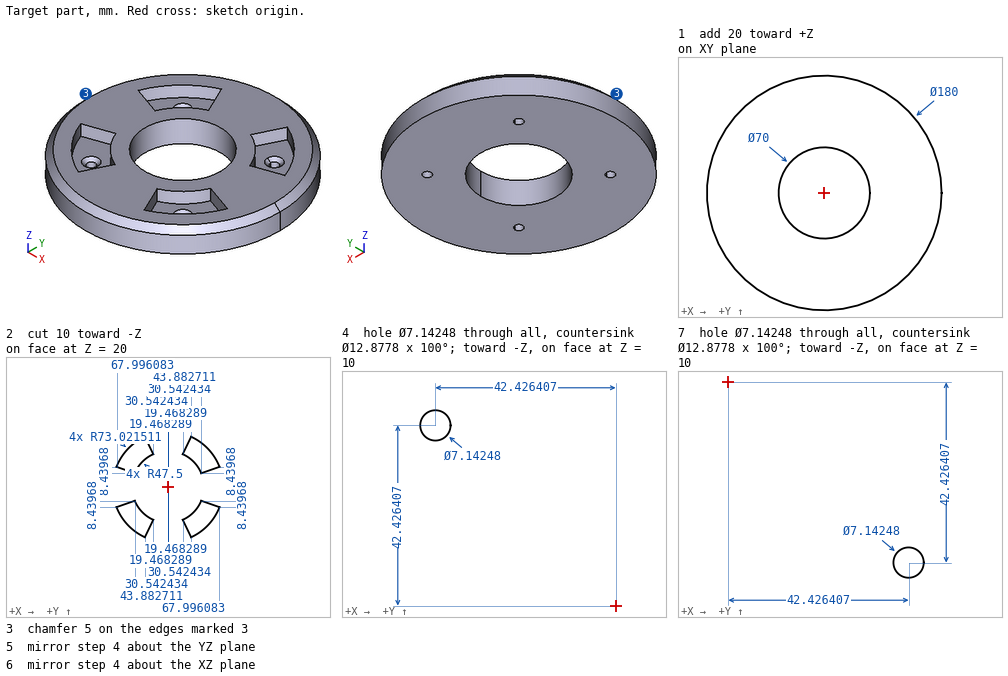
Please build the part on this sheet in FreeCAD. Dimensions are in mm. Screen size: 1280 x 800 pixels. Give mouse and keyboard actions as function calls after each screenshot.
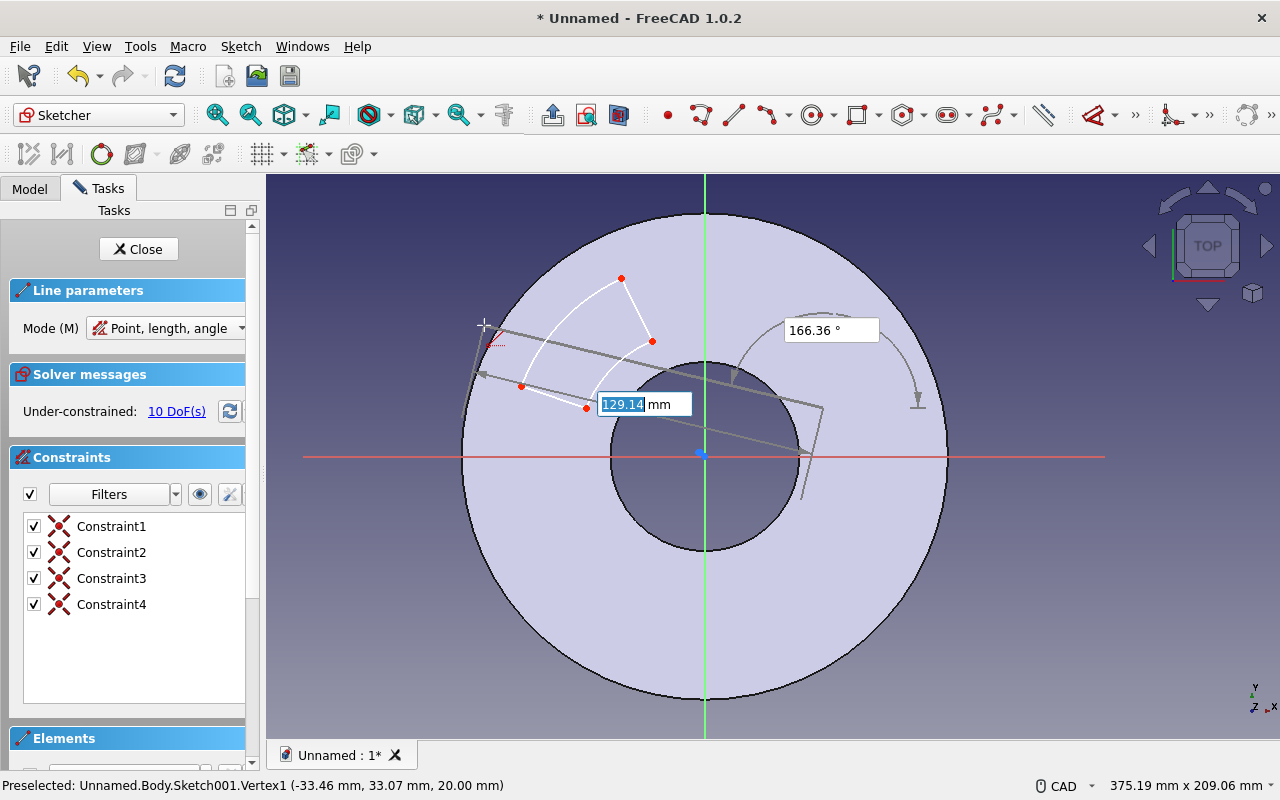
click(889, 385)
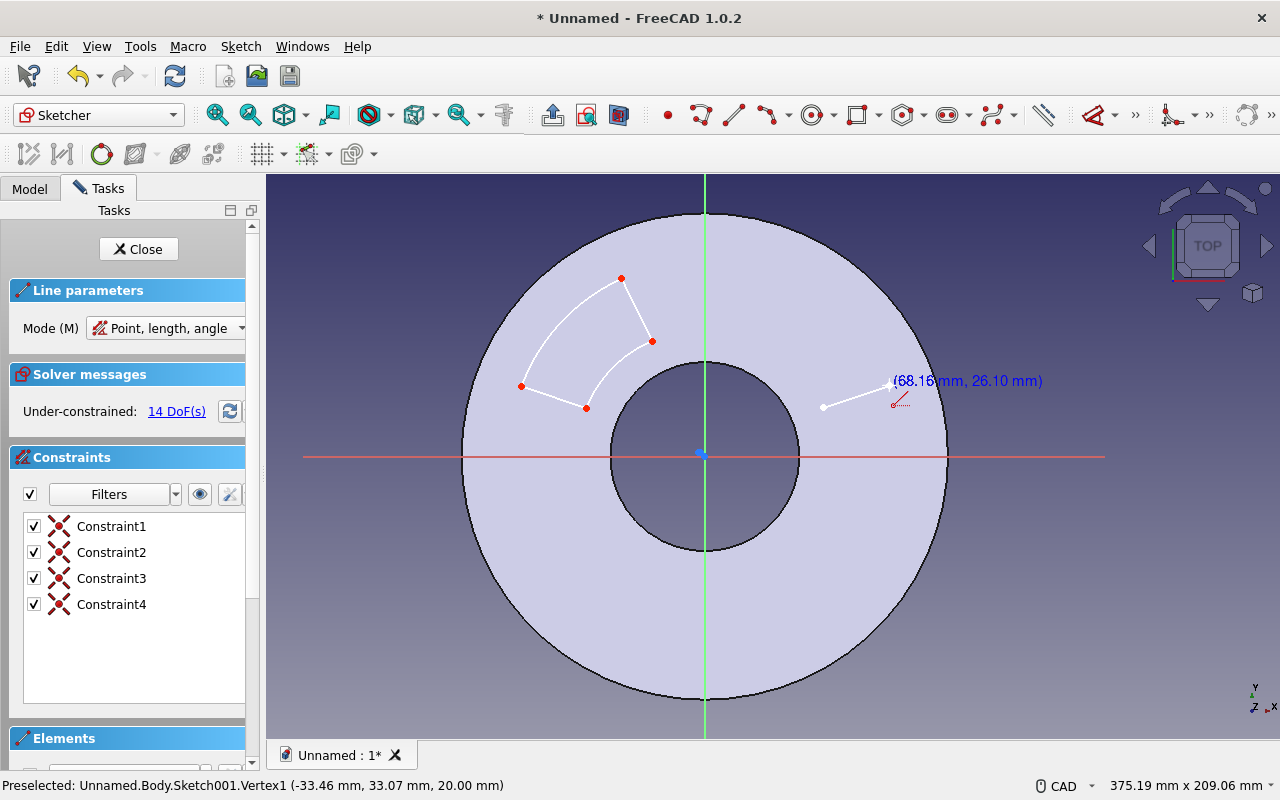
click(787, 277)
click(757, 339)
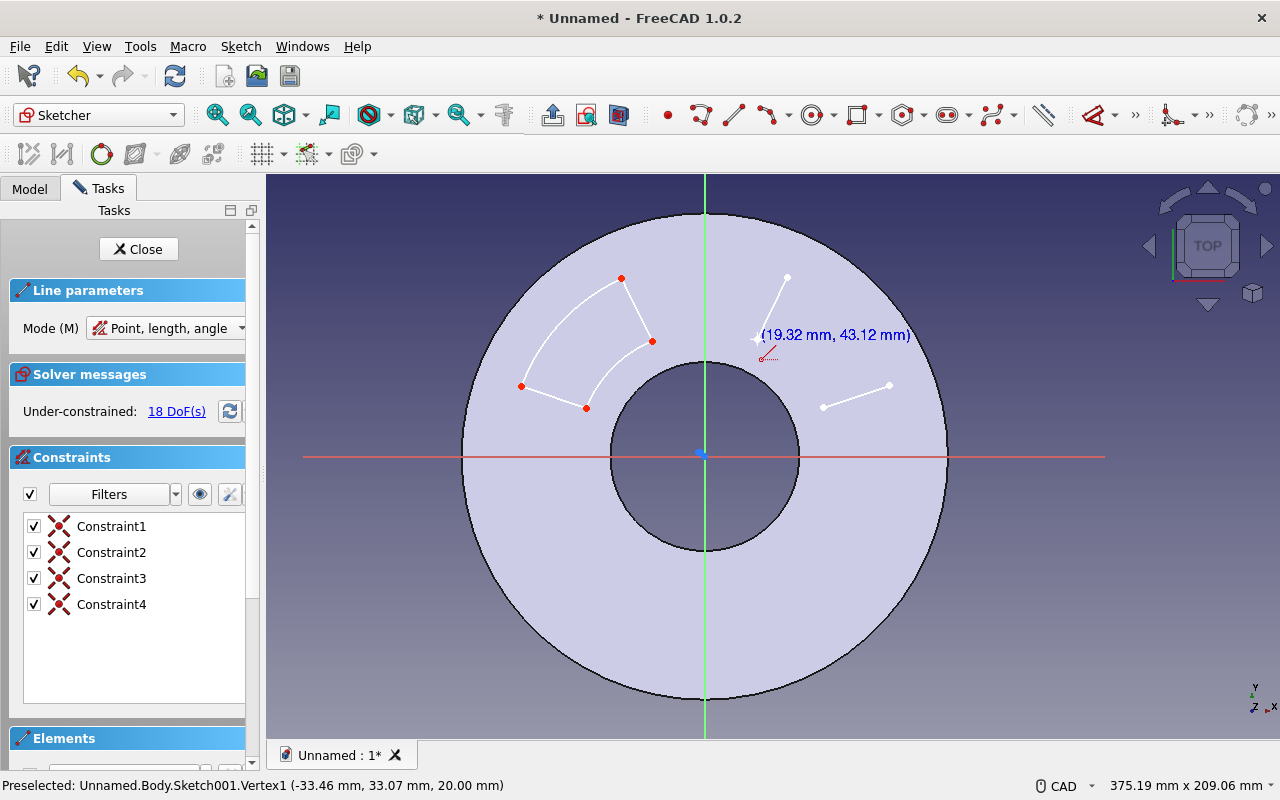
click(766, 116)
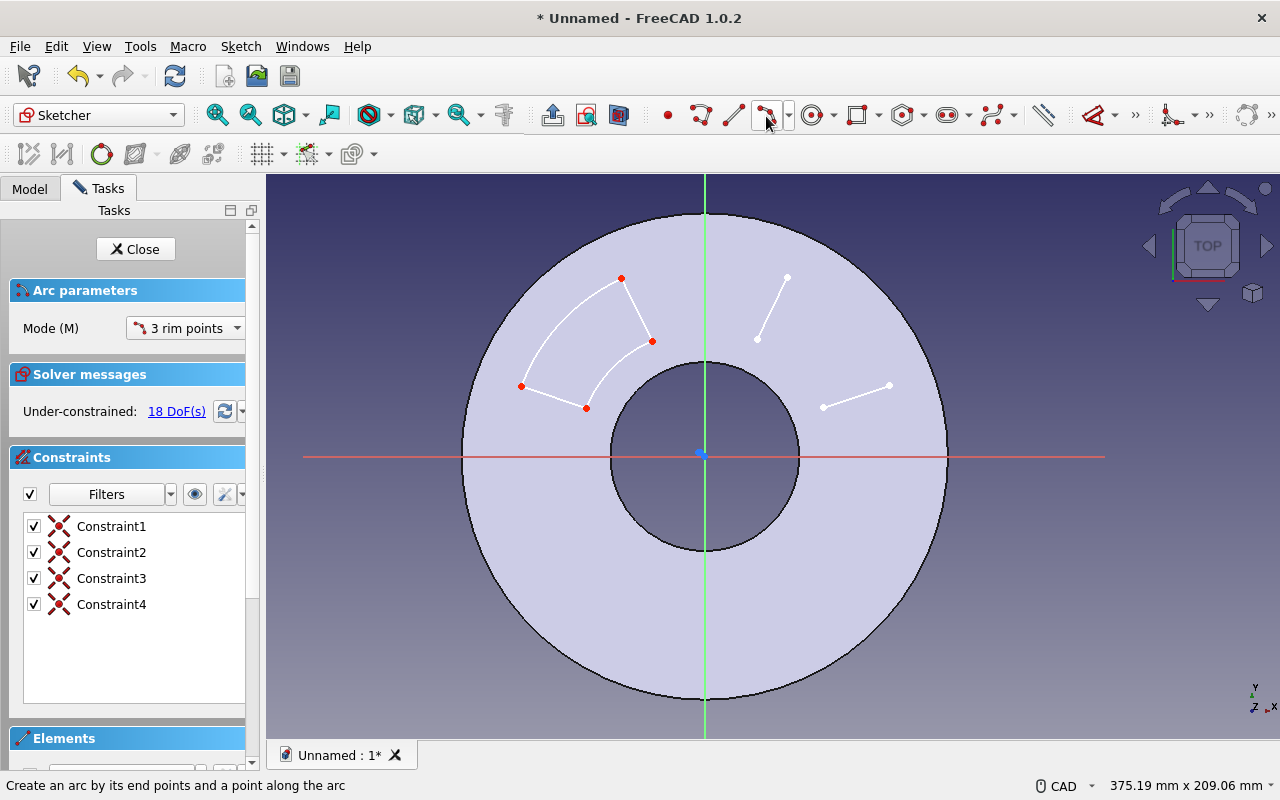
click(889, 386)
click(787, 278)
click(848, 321)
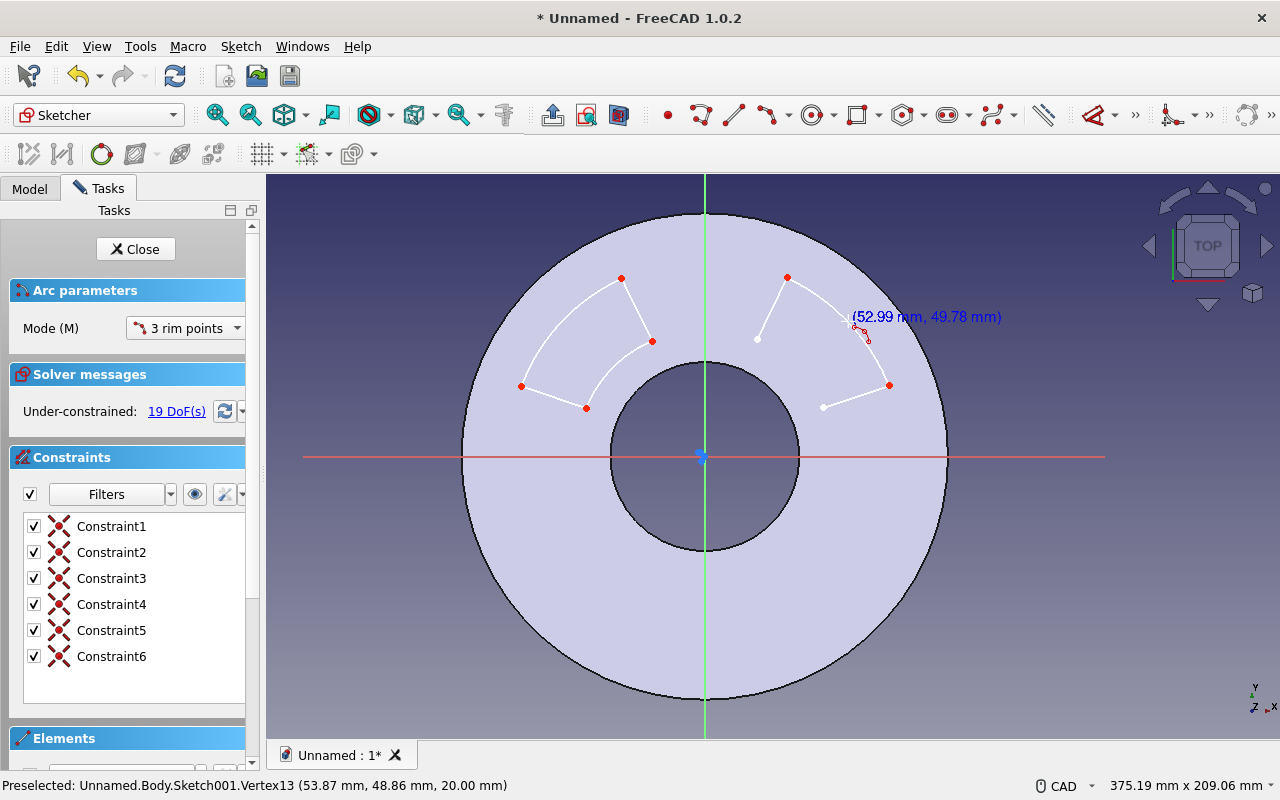
click(757, 340)
click(823, 408)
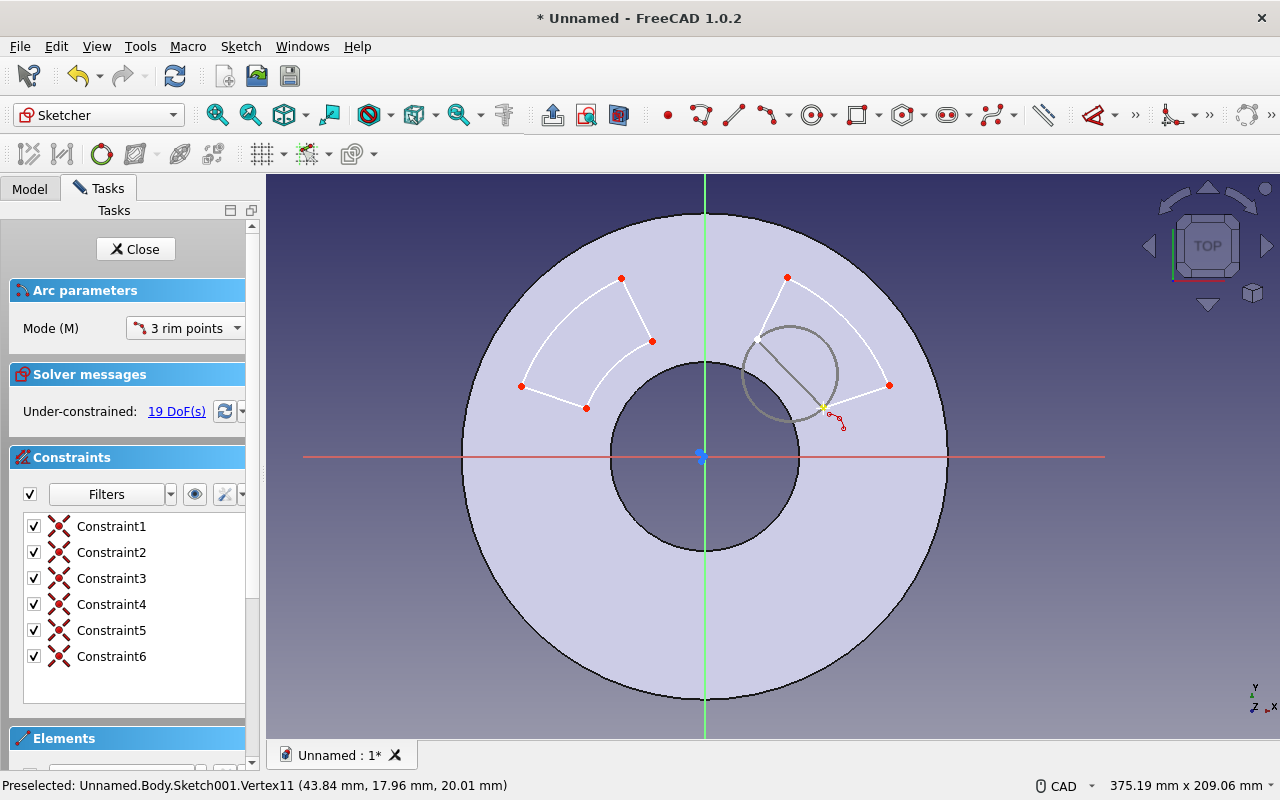
scroll(797, 367, up, 3)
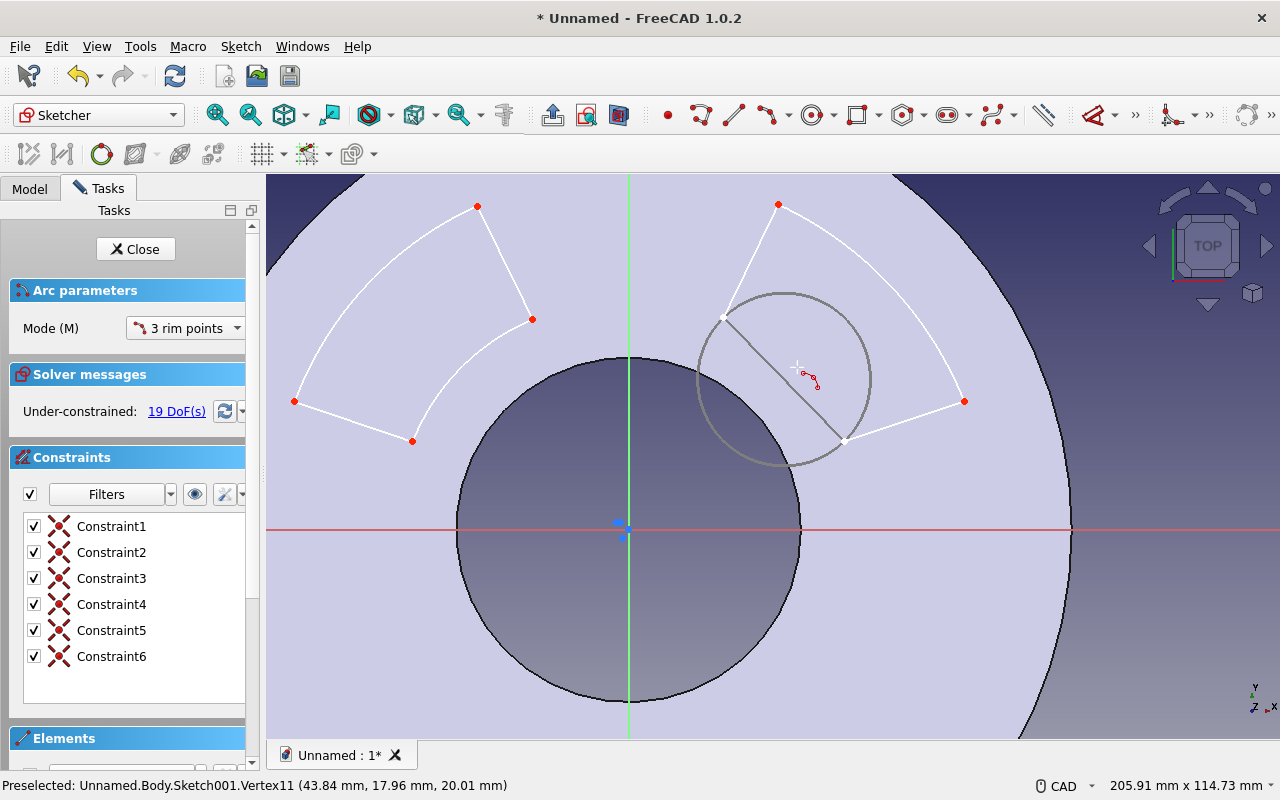
click(796, 367)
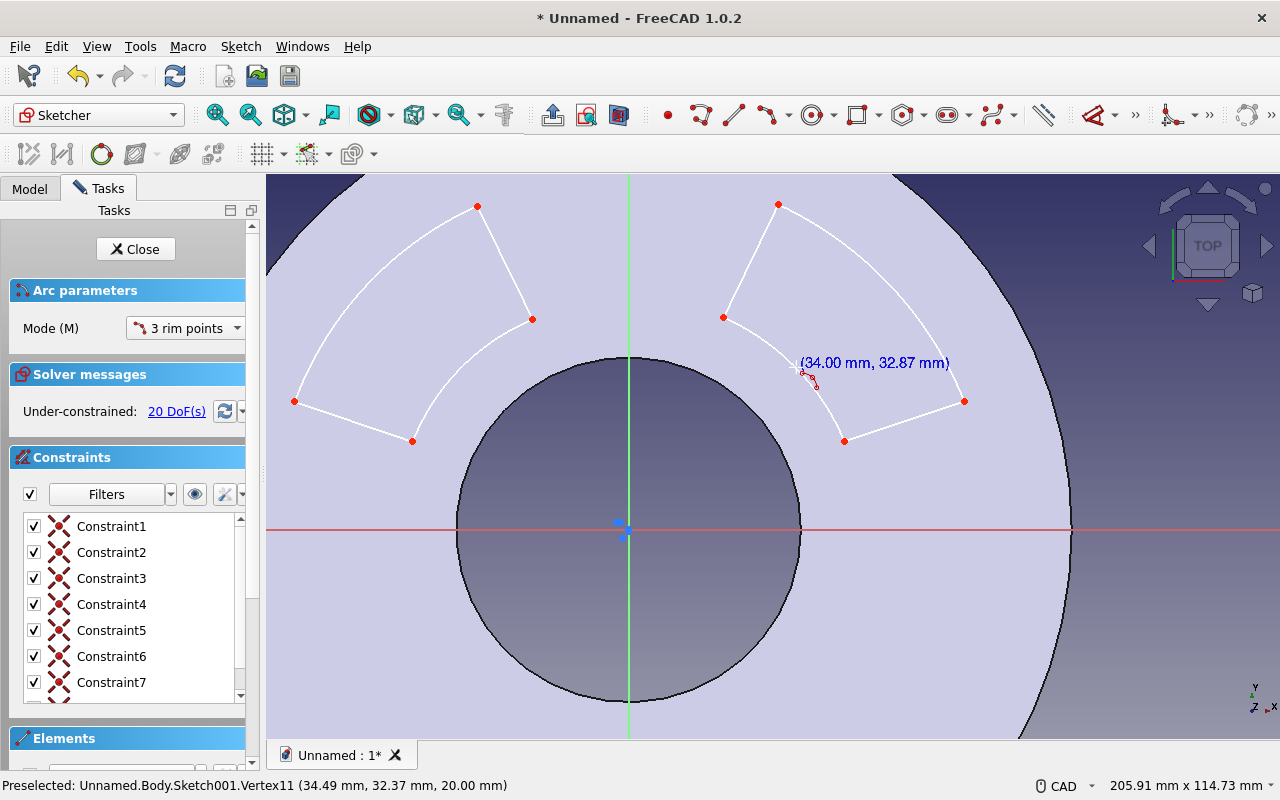
click(734, 116)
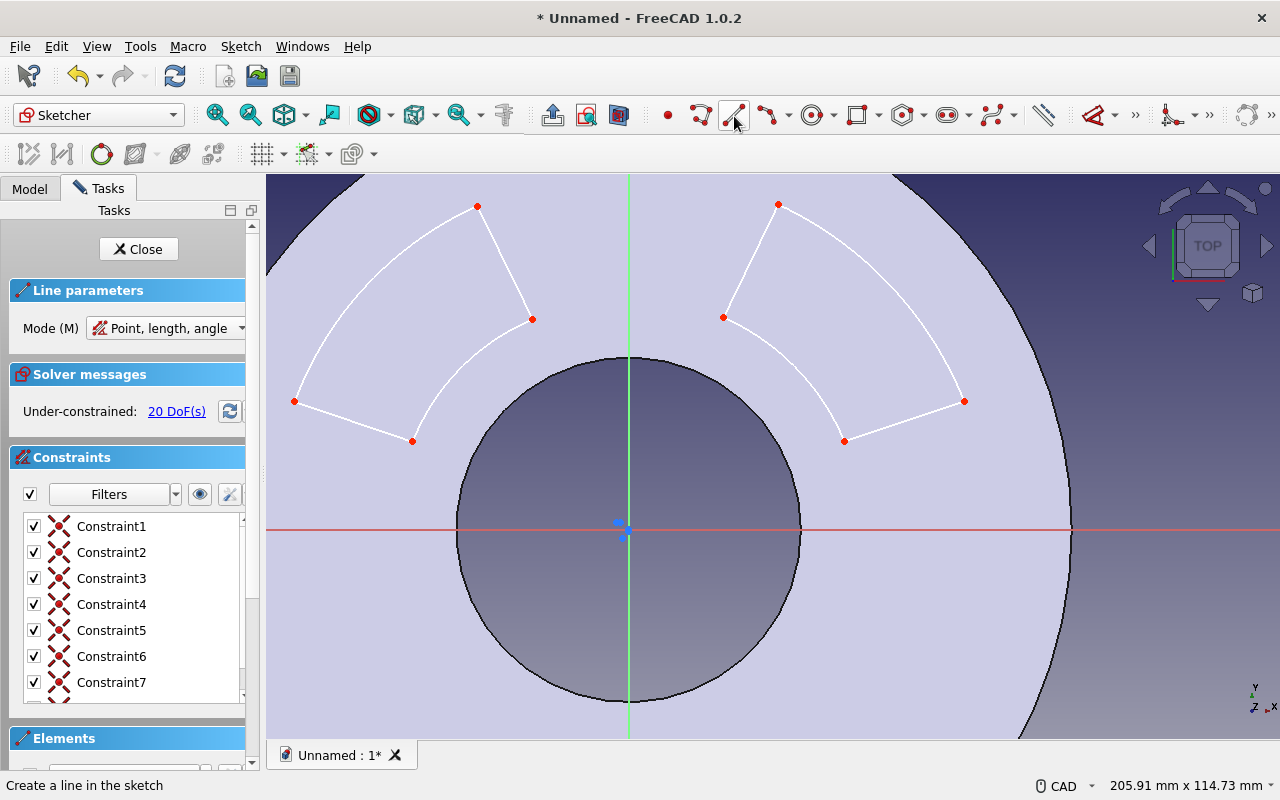
scroll(797, 367, down, 3)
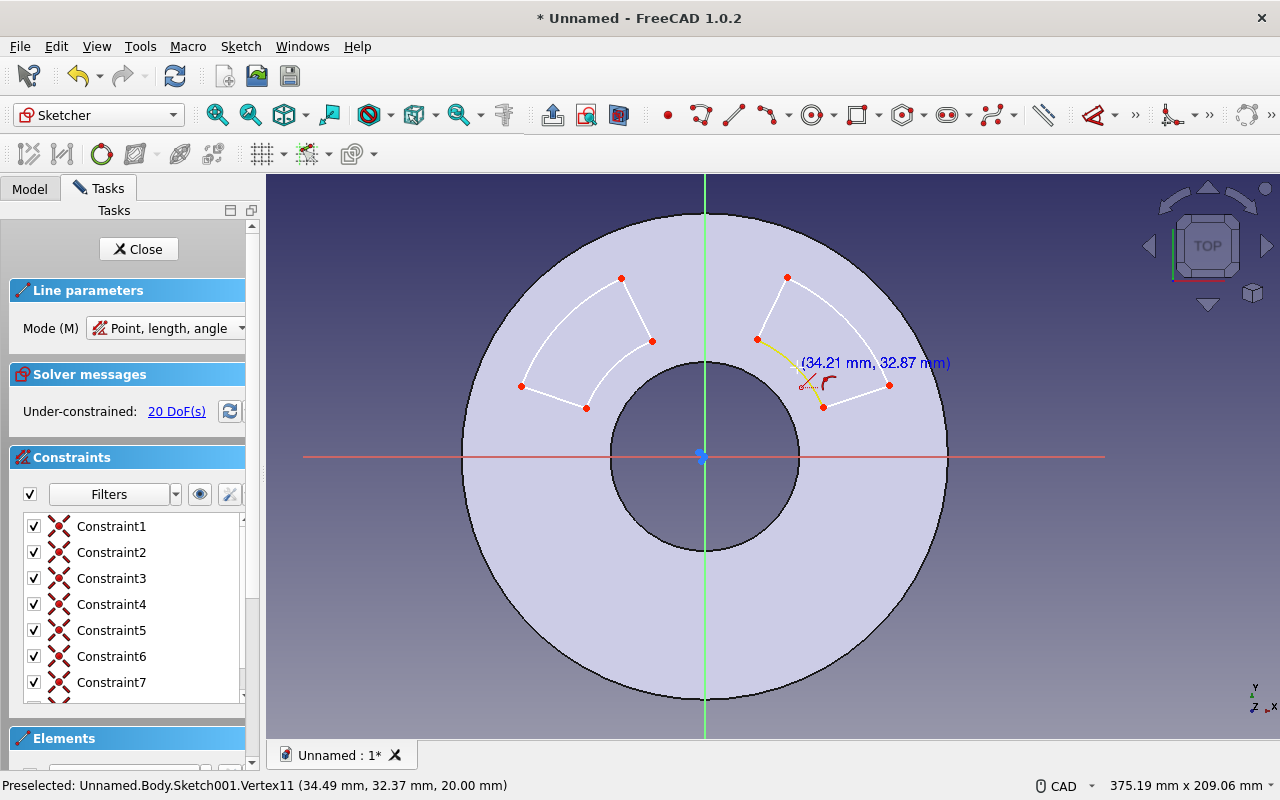
click(757, 574)
click(787, 636)